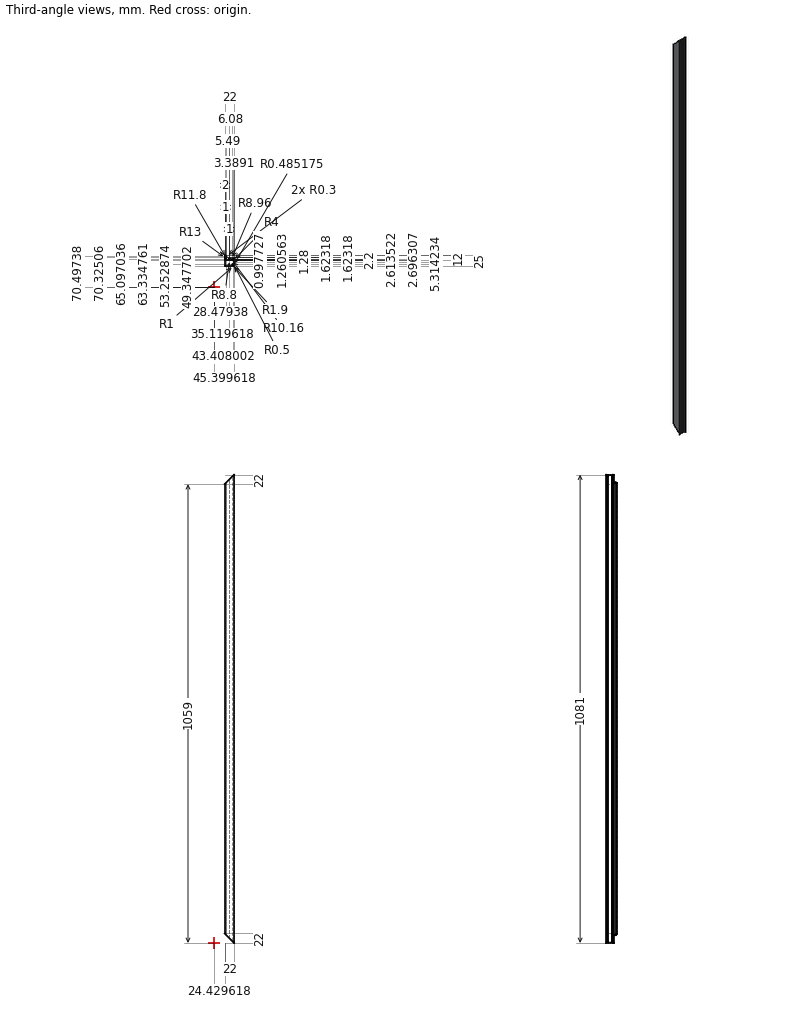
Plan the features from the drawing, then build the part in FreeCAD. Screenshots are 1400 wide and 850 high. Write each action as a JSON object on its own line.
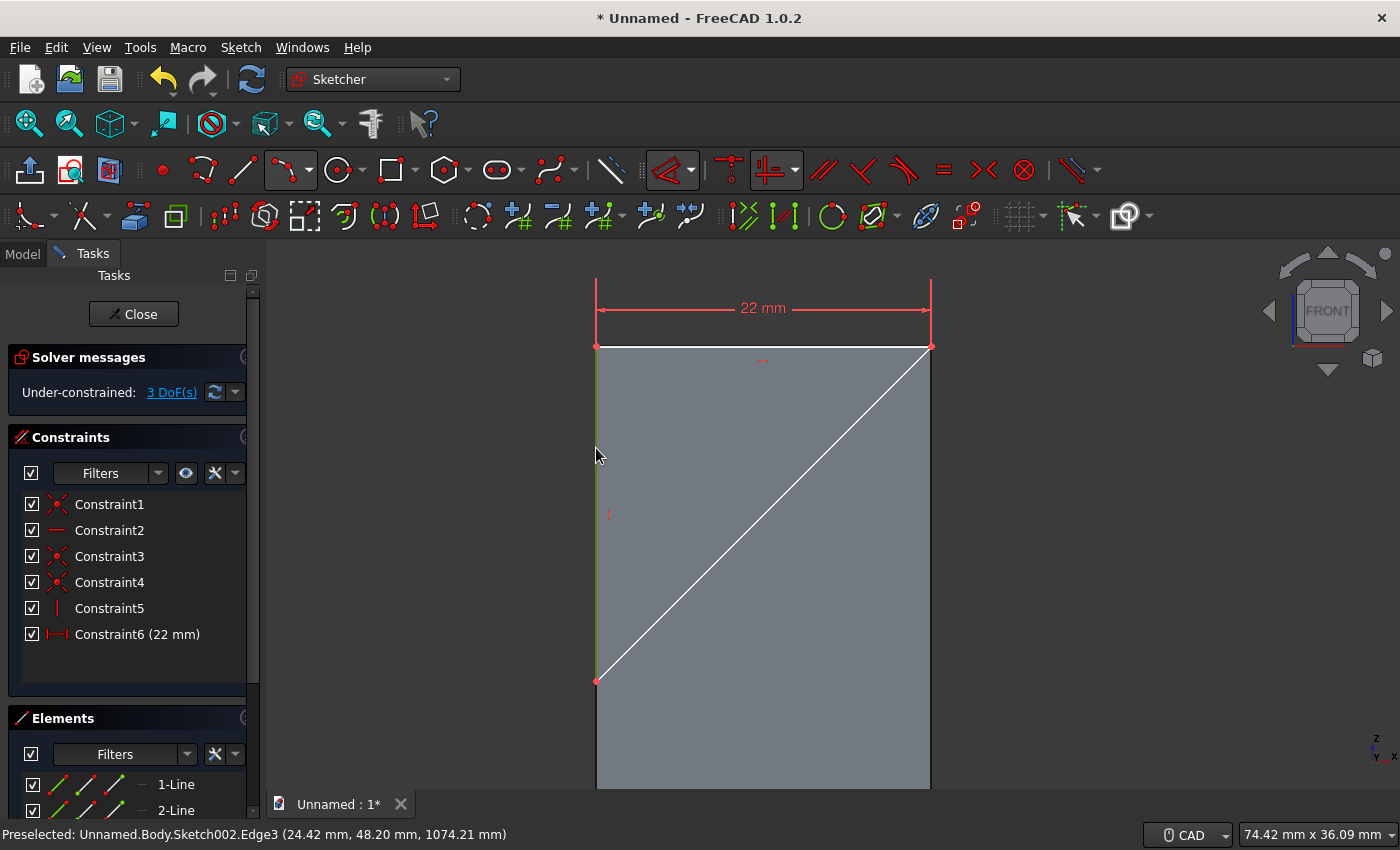
{"action": "left_click", "coordinate": [694, 170]}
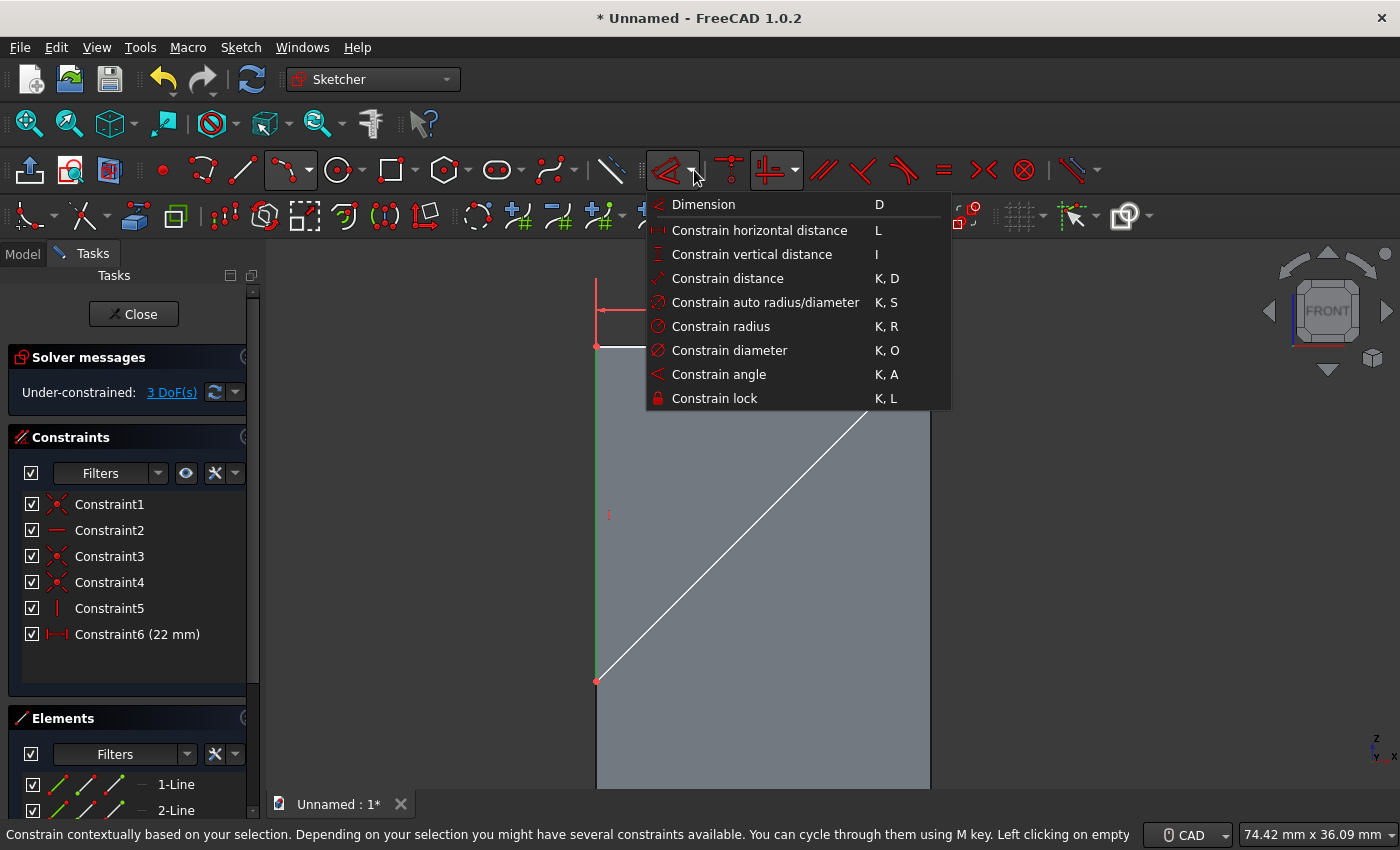
{"action": "left_click", "coordinate": [799, 254]}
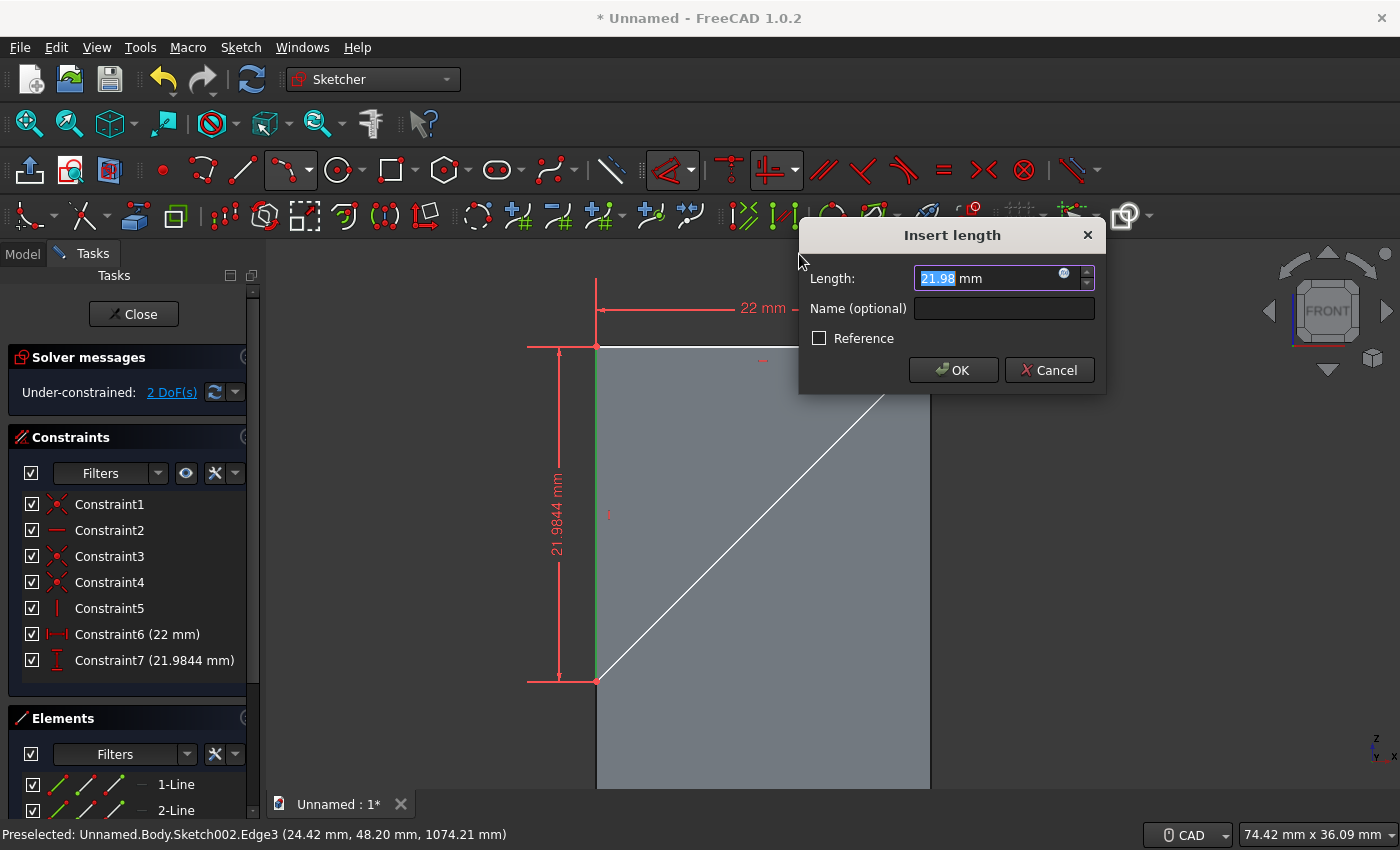
{"action": "type", "text": "22"}
{"action": "key", "text": "Return"}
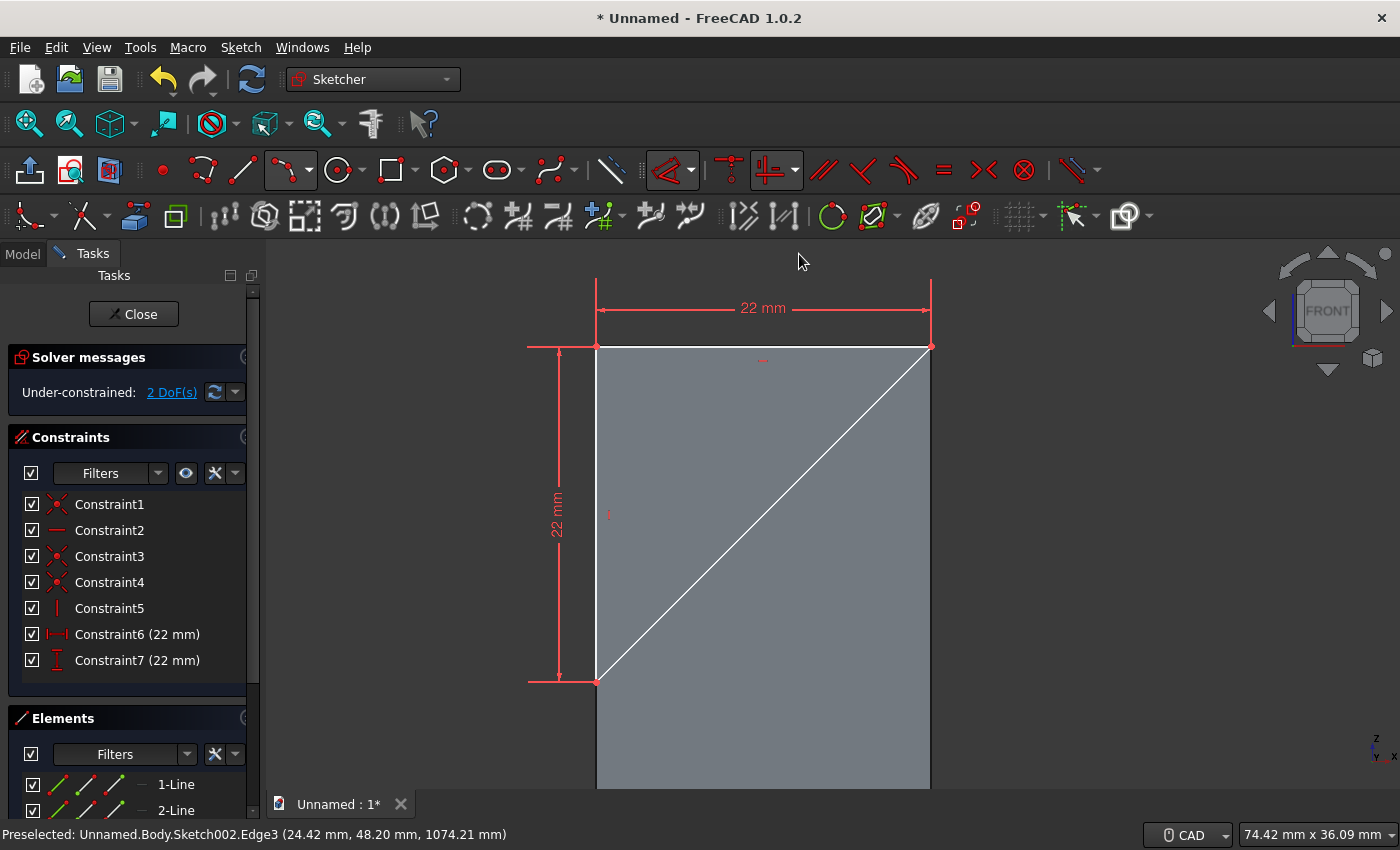
{"action": "left_click", "coordinate": [596, 682]}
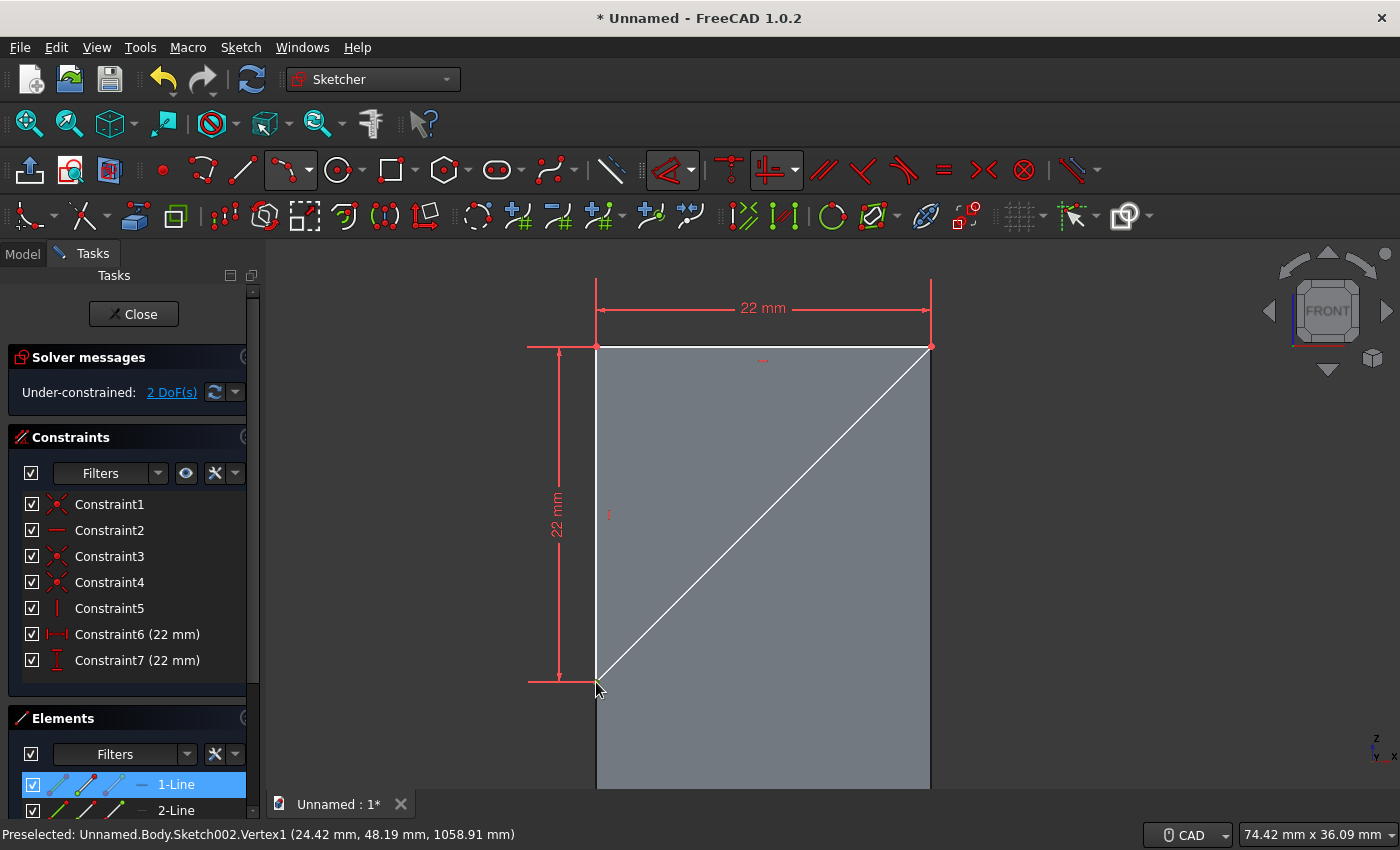
{"action": "key", "text": "i"}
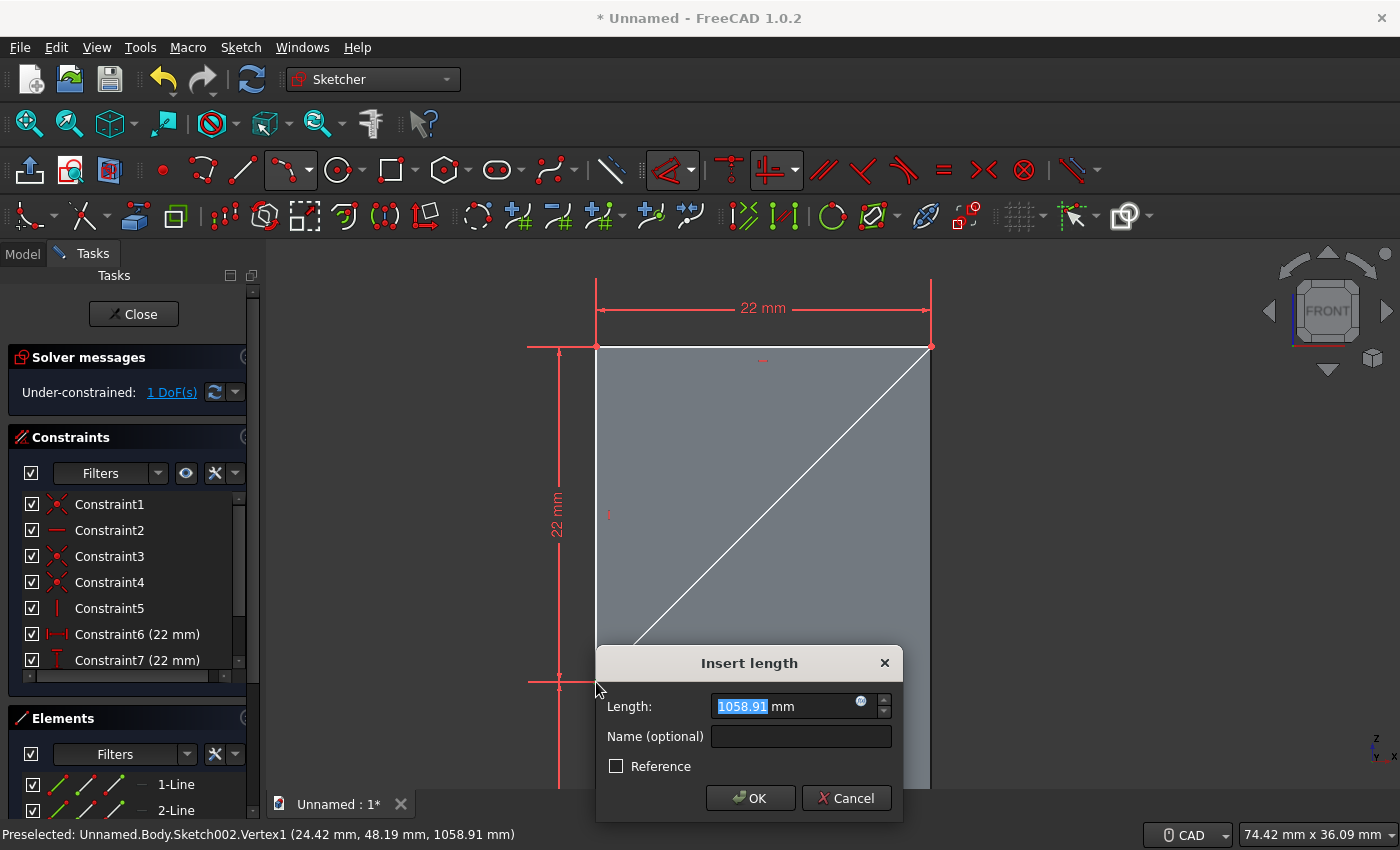
{"action": "type", "text": "1059"}
{"action": "key", "text": "Return"}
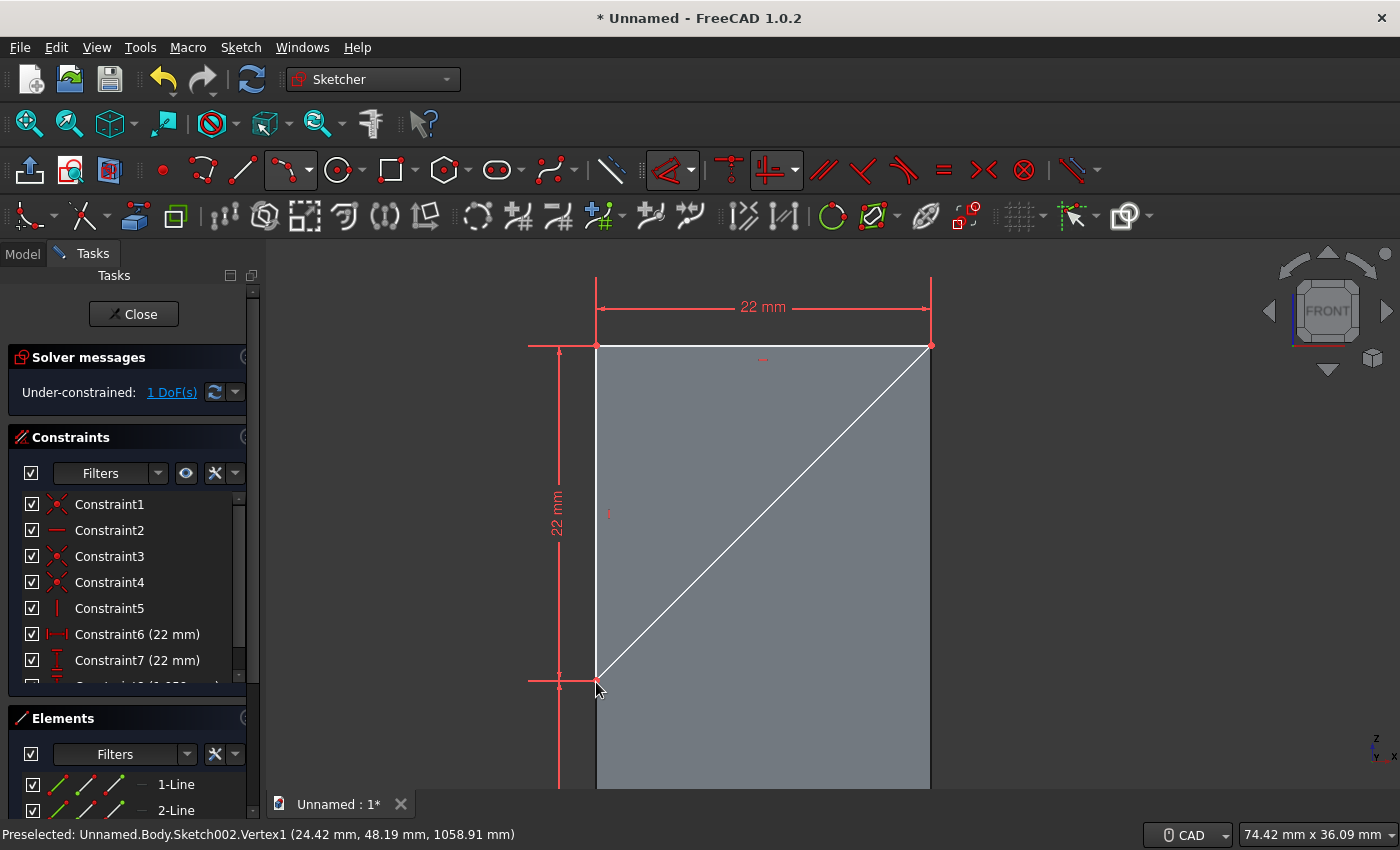
{"action": "left_click", "coordinate": [596, 681]}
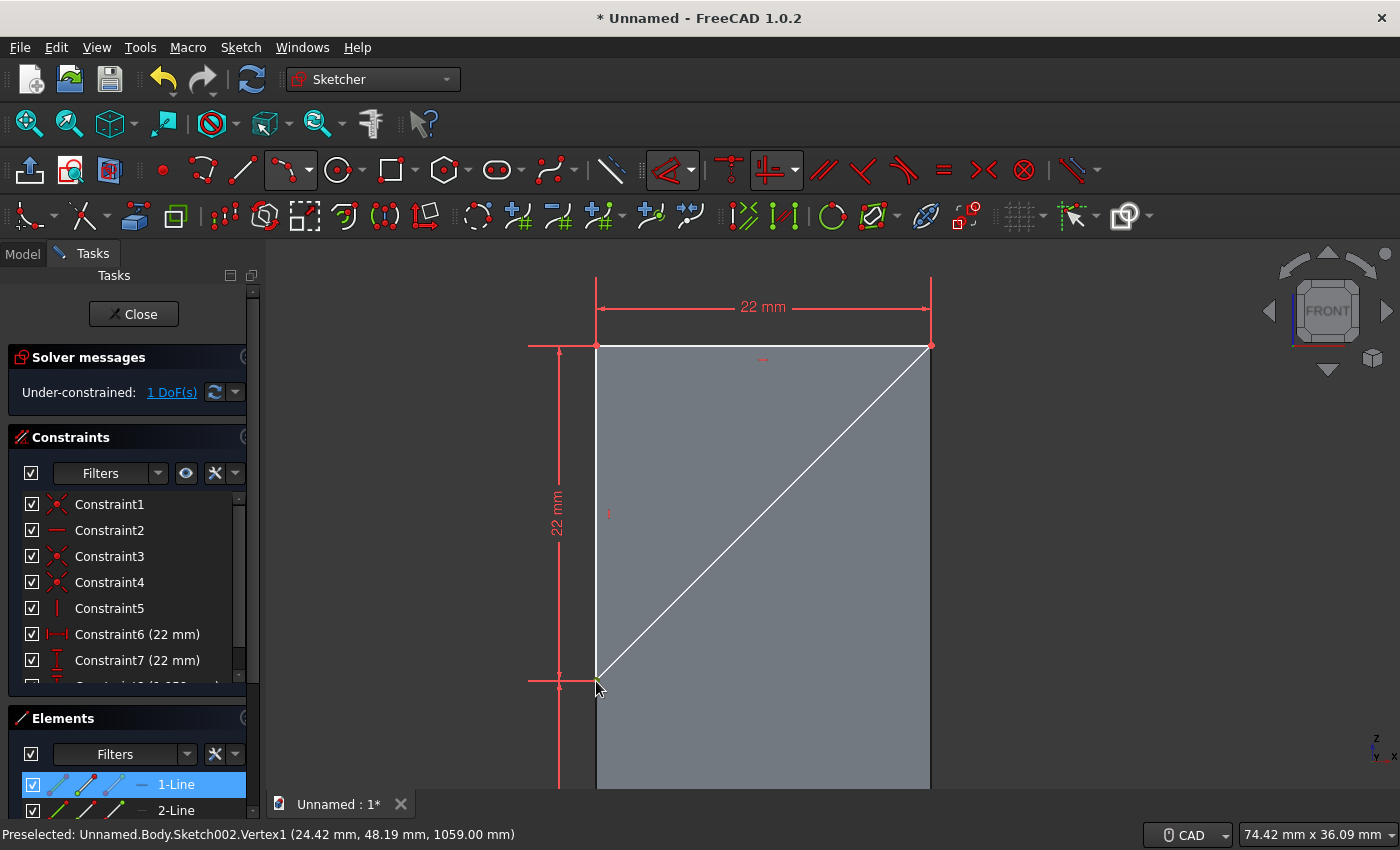
{"action": "key", "text": "l"}